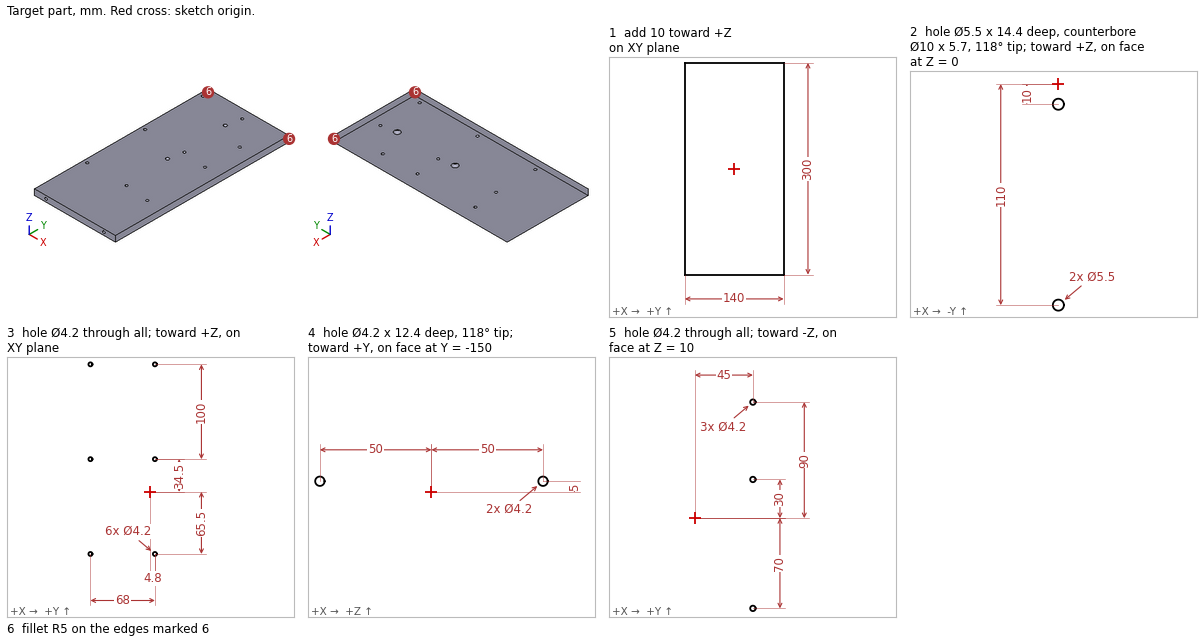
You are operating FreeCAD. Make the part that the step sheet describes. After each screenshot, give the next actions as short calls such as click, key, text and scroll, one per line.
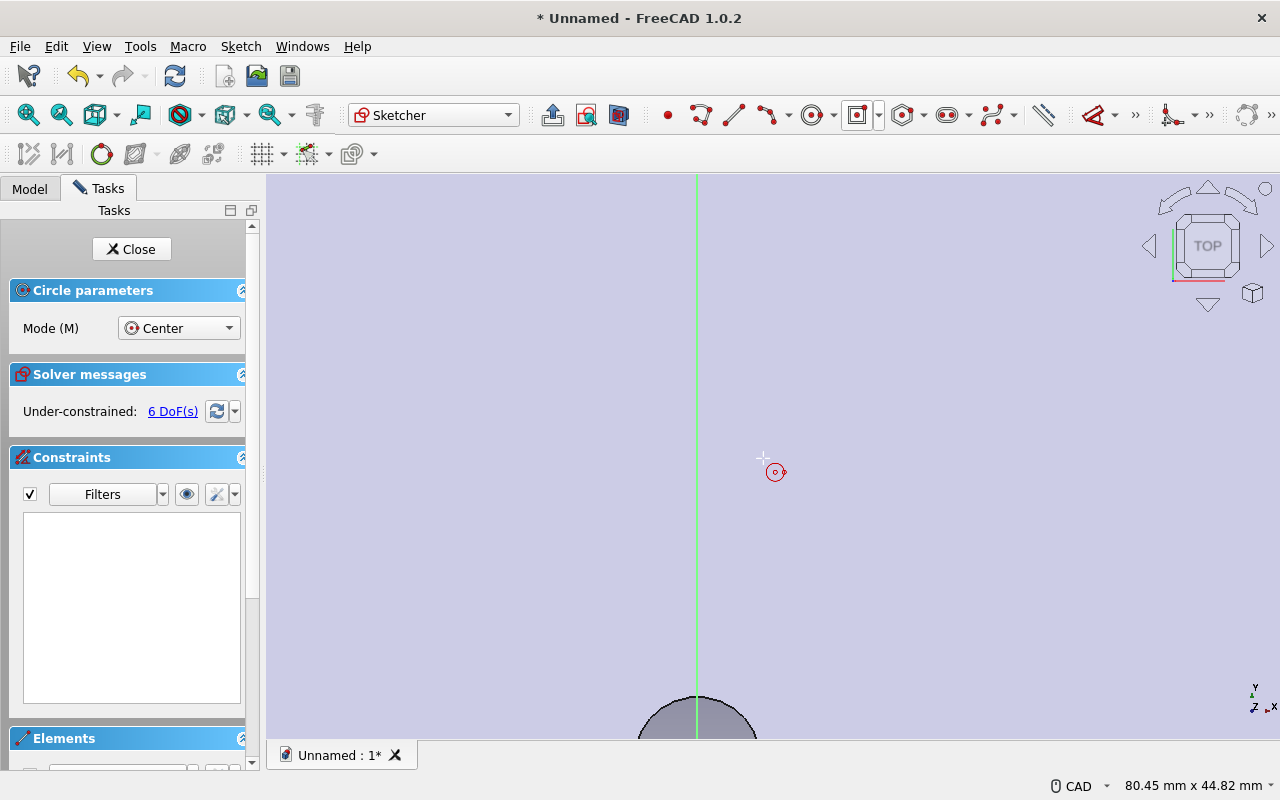
scroll(763, 457, down, 10)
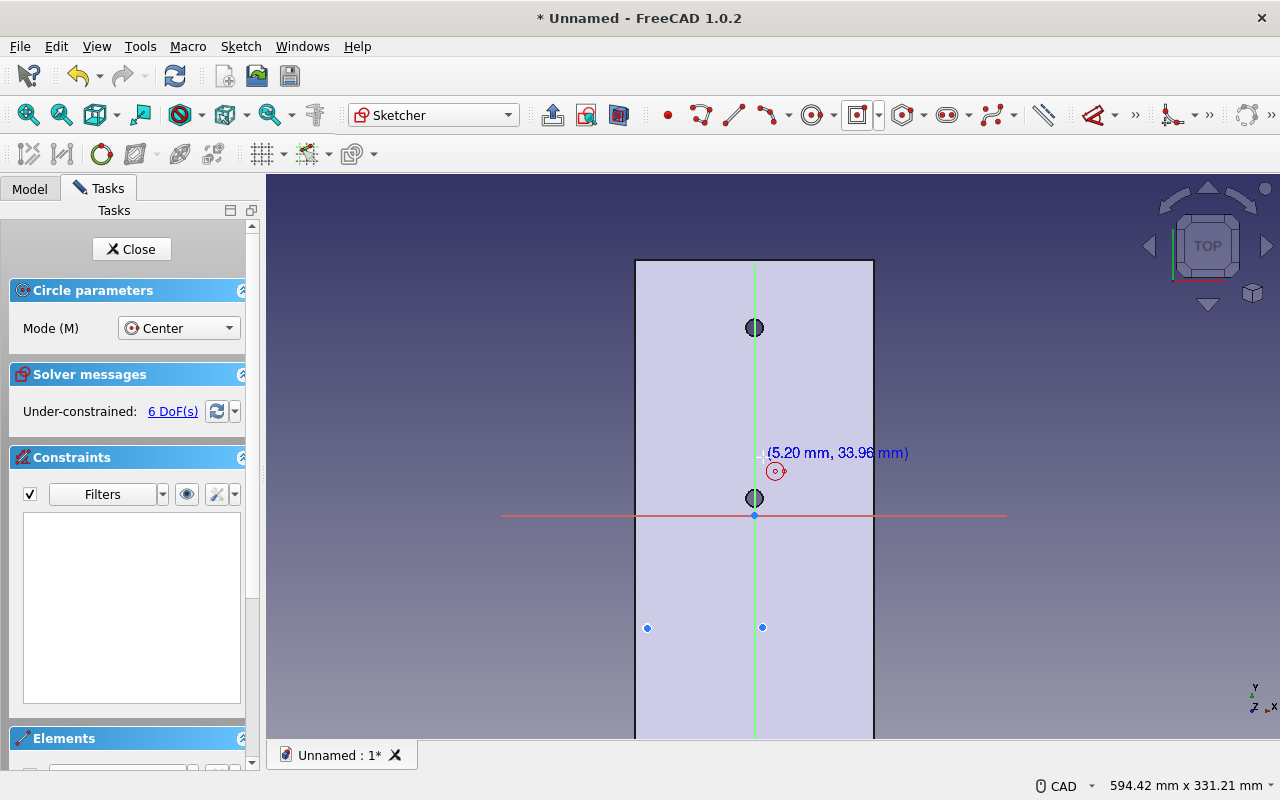
scroll(763, 457, up, 4)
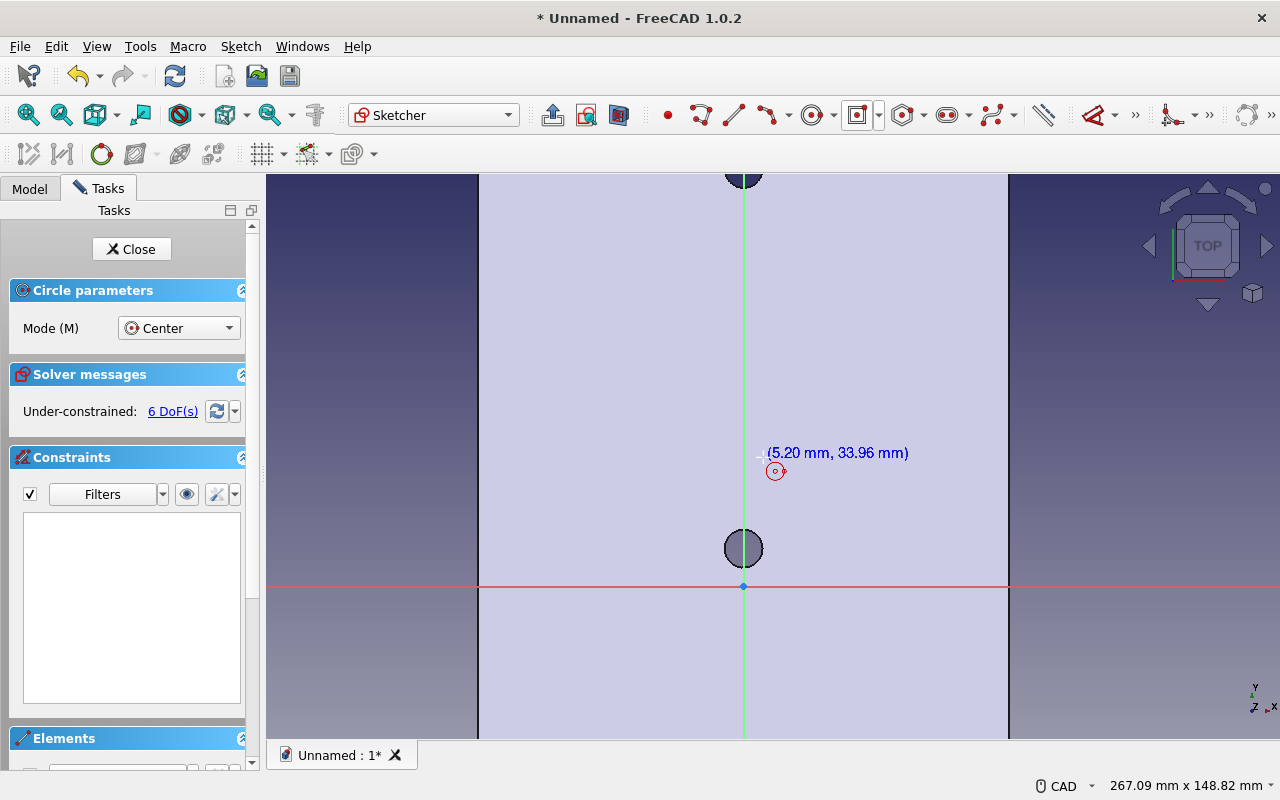
click(762, 456)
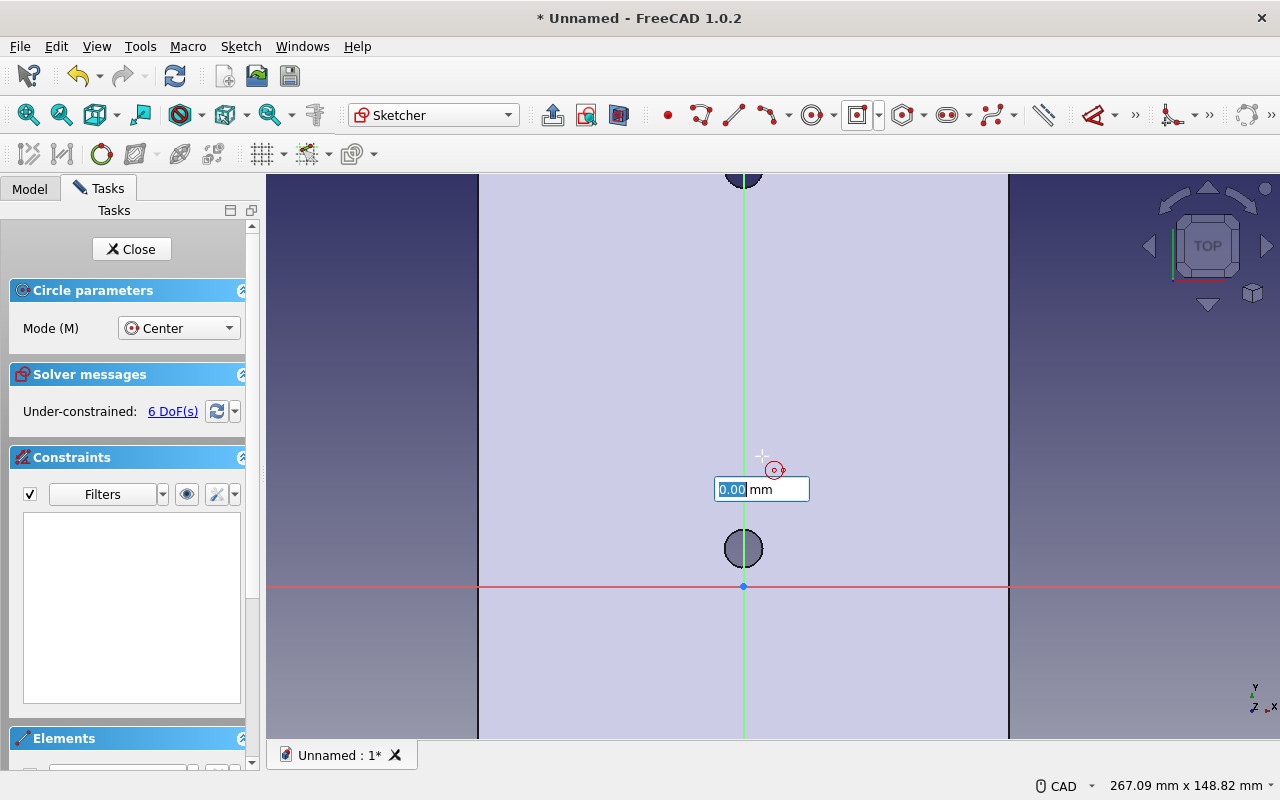
scroll(767, 450, up, 4)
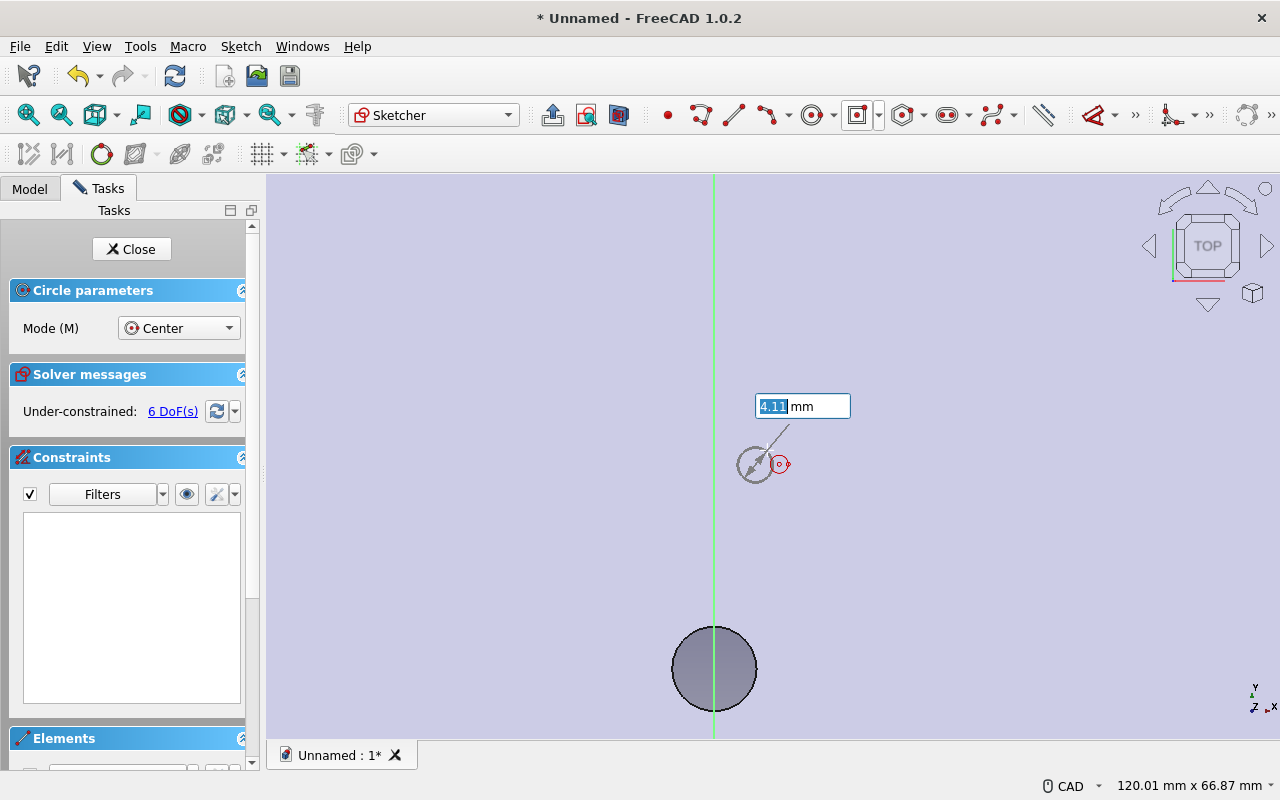
click(767, 449)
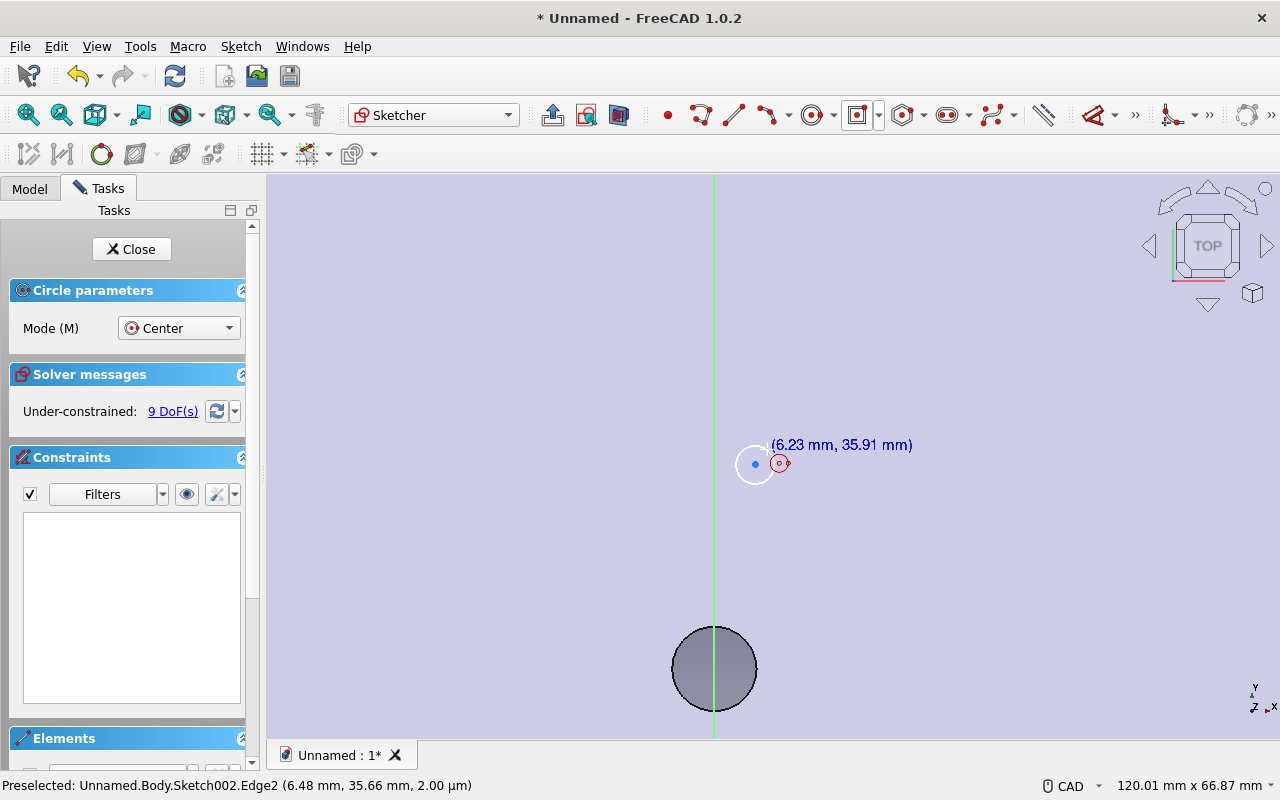
scroll(764, 455, down, 8)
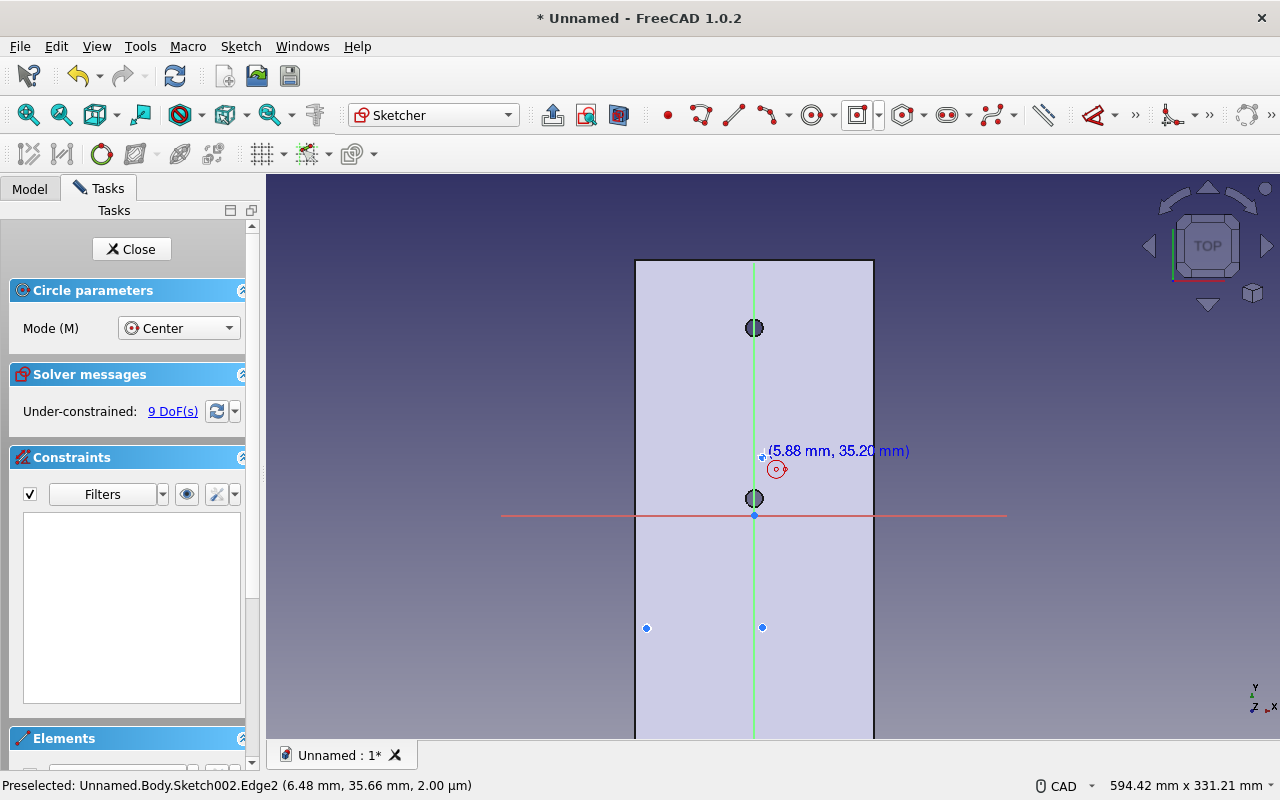
scroll(647, 457, up, 10)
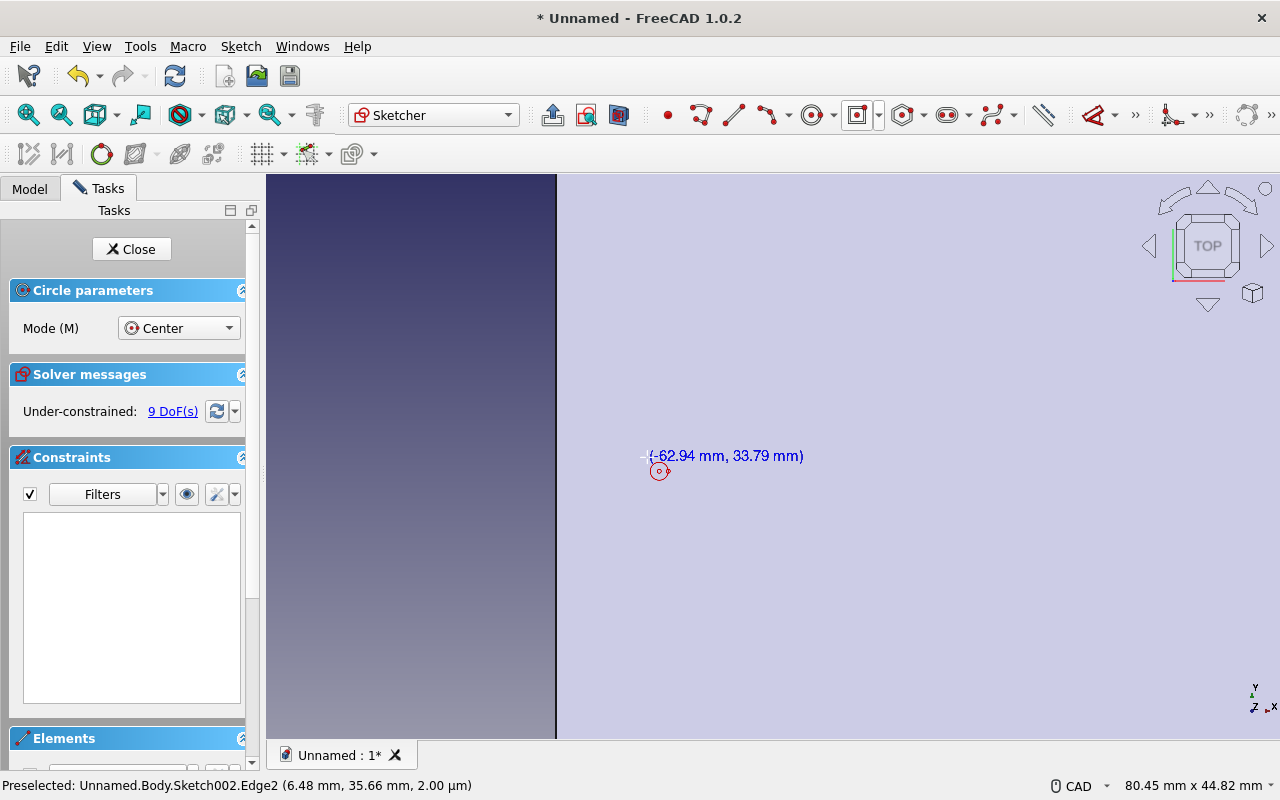
scroll(647, 457, down, 10)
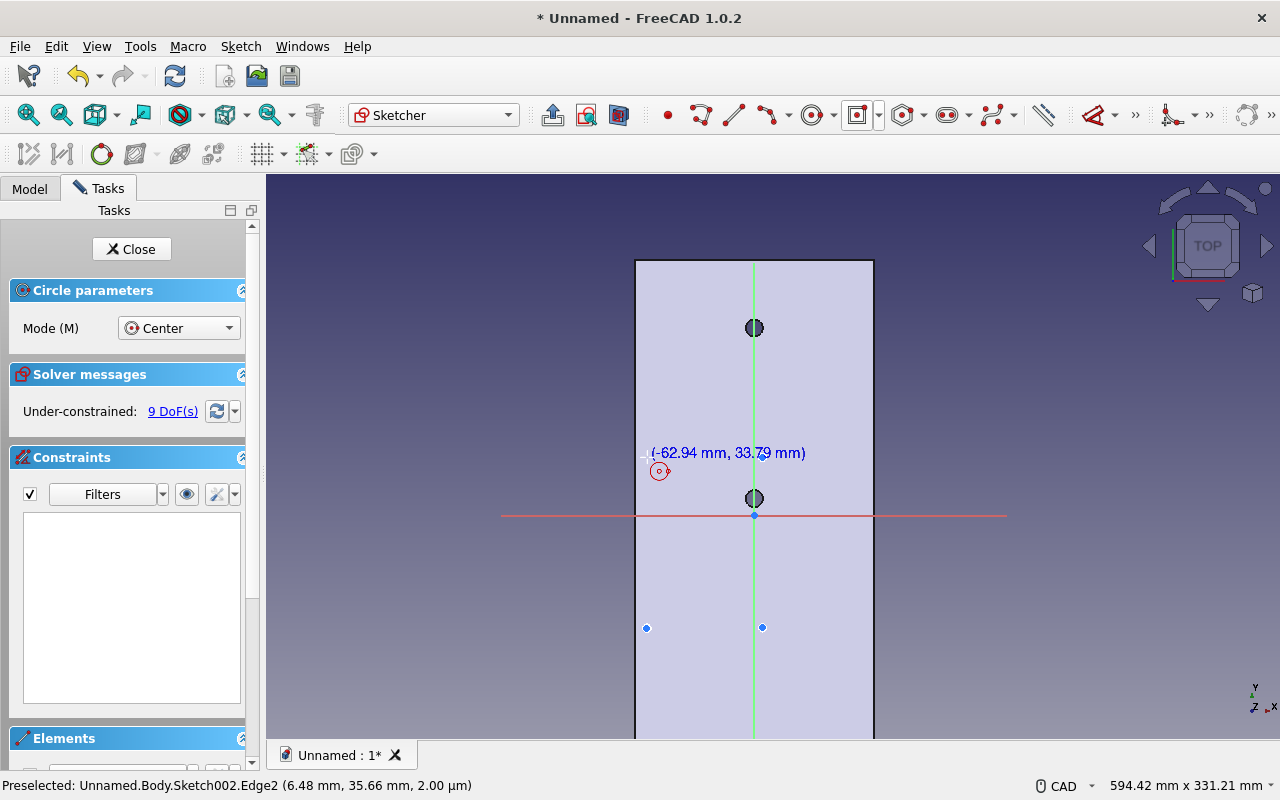
click(647, 457)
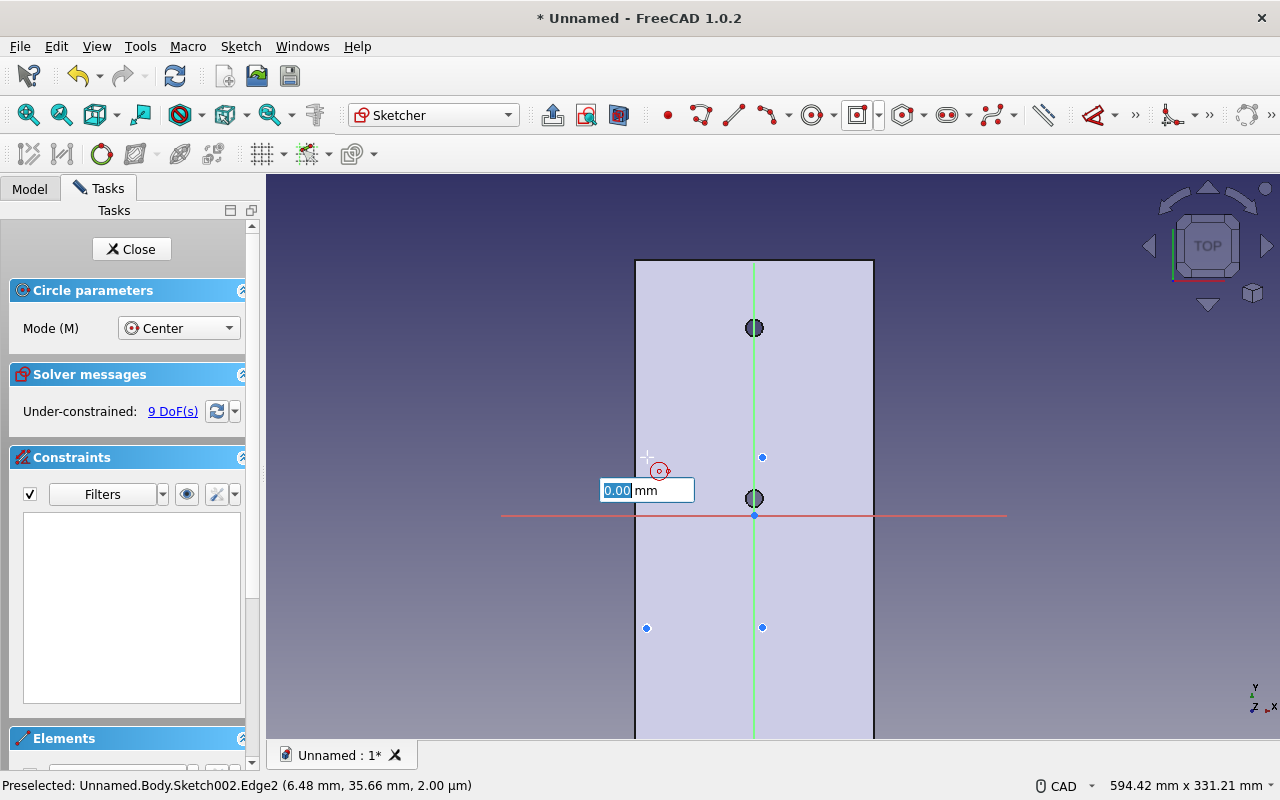
scroll(649, 454, up, 8)